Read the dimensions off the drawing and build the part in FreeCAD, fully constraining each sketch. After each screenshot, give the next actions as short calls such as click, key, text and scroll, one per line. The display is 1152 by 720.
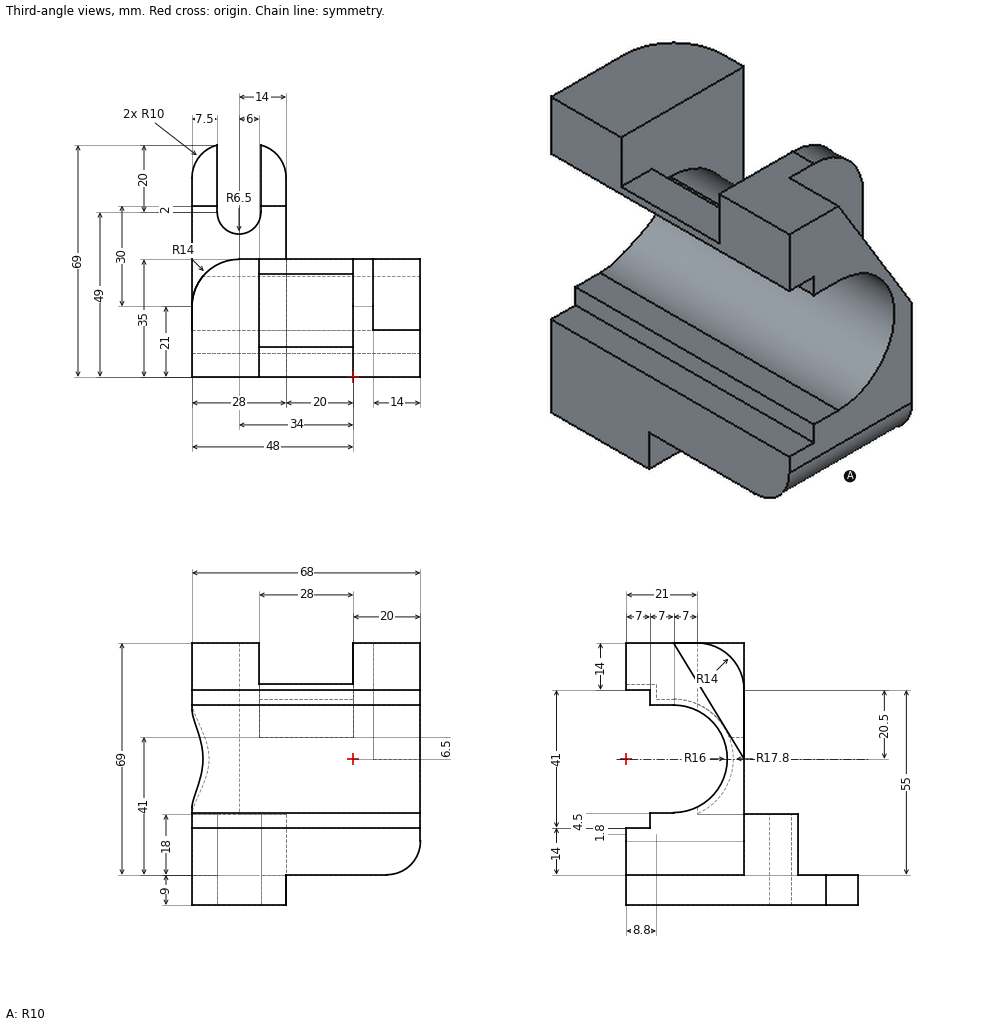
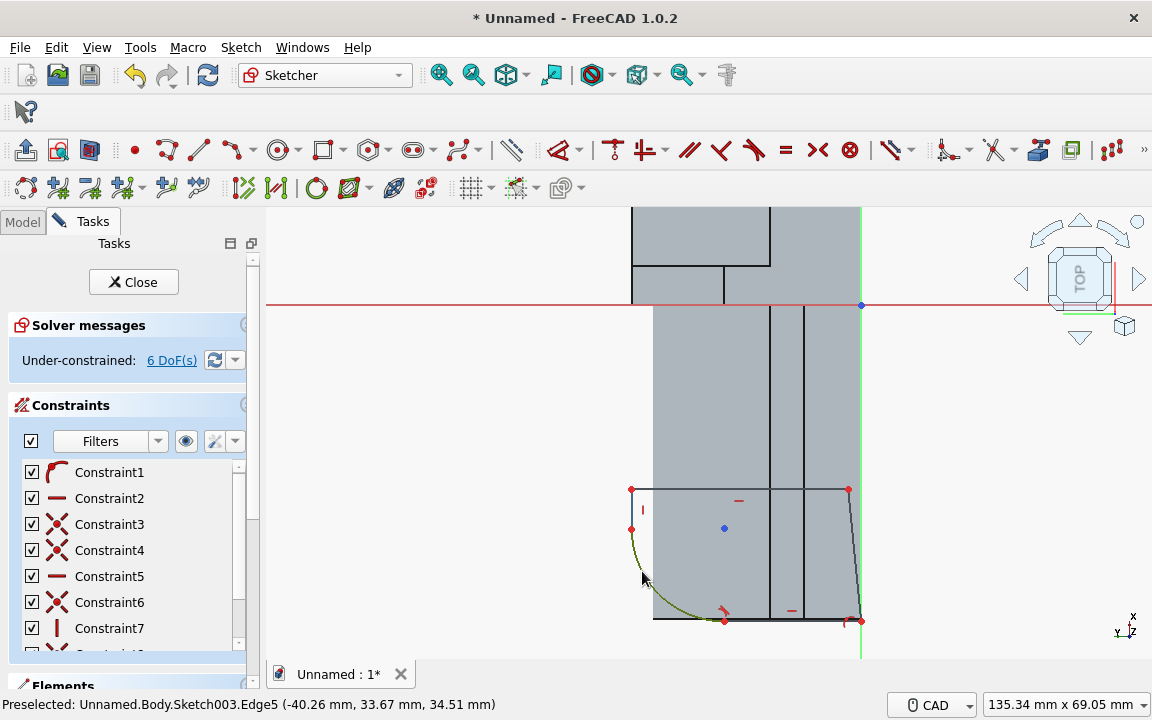
click(754, 150)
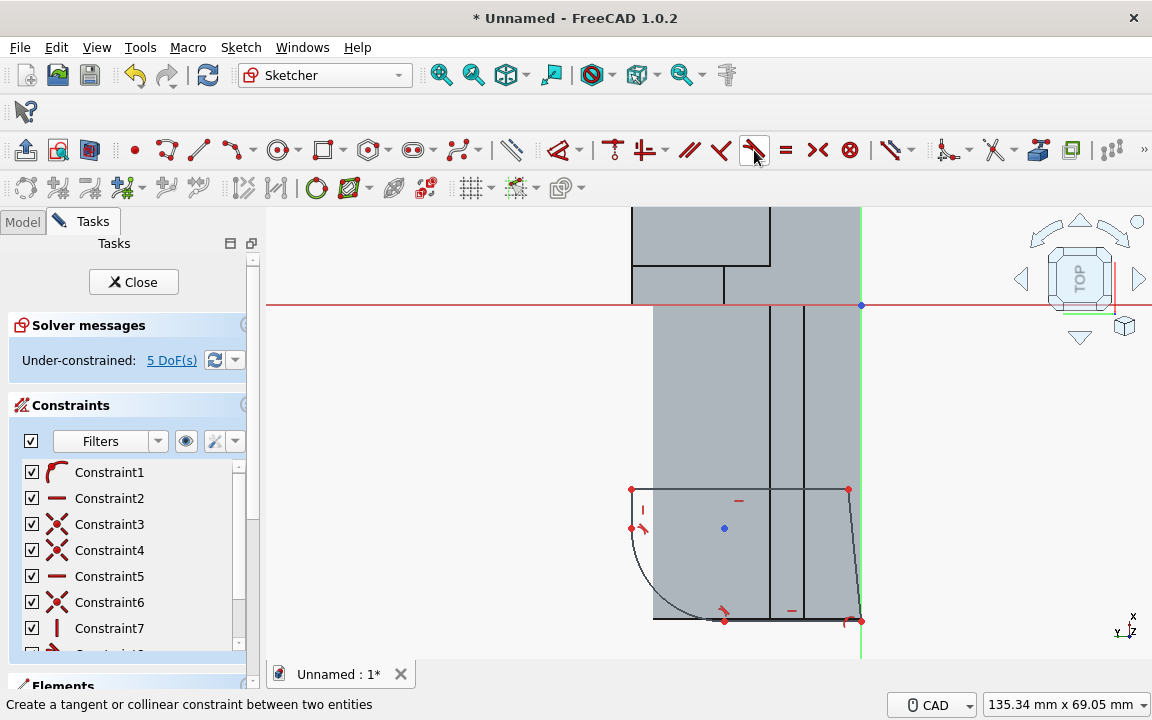
click(857, 582)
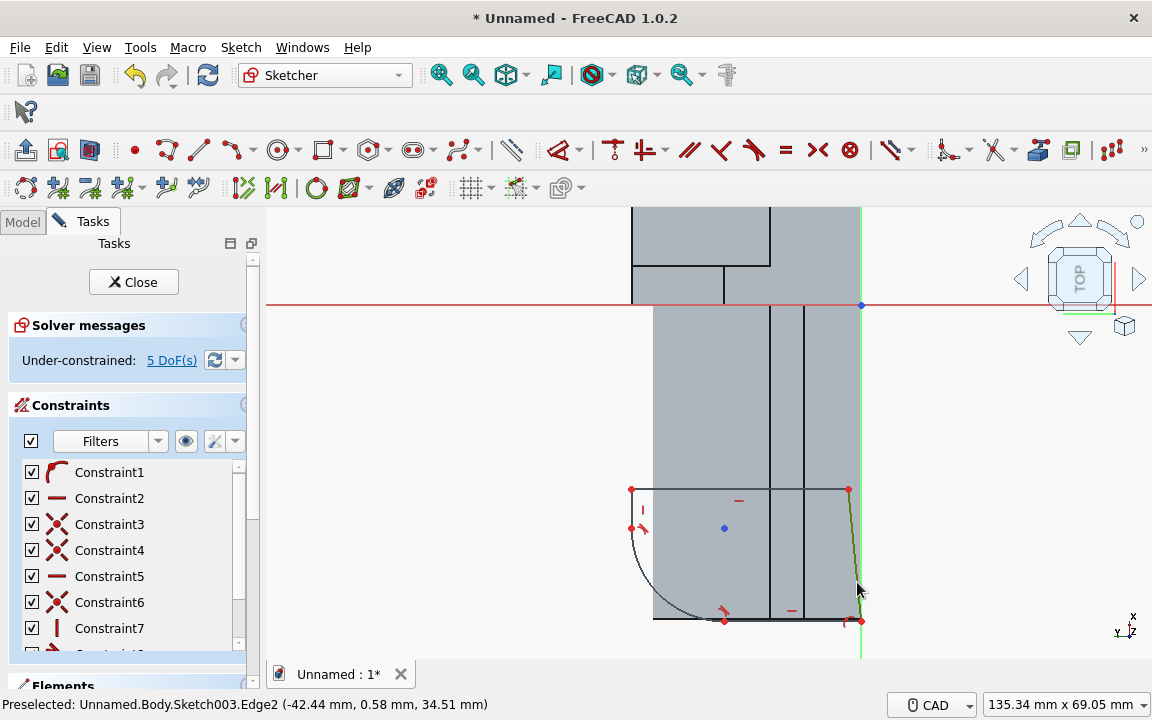
key(v)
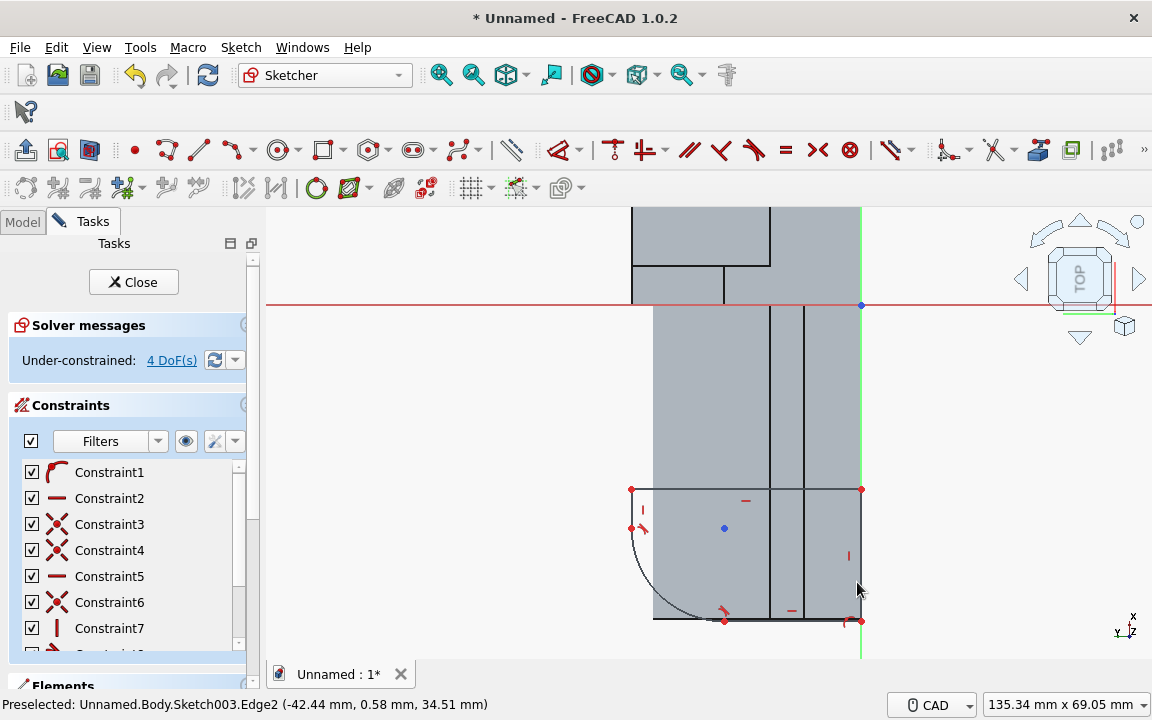
click(558, 150)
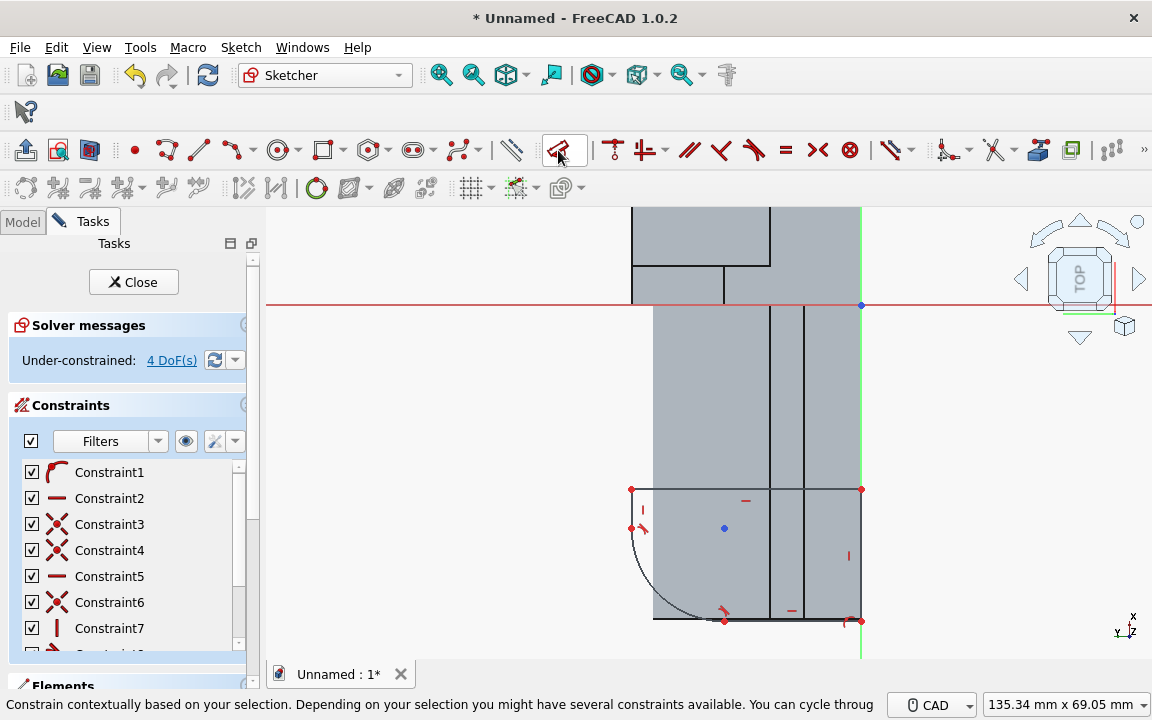
click(642, 571)
click(614, 586)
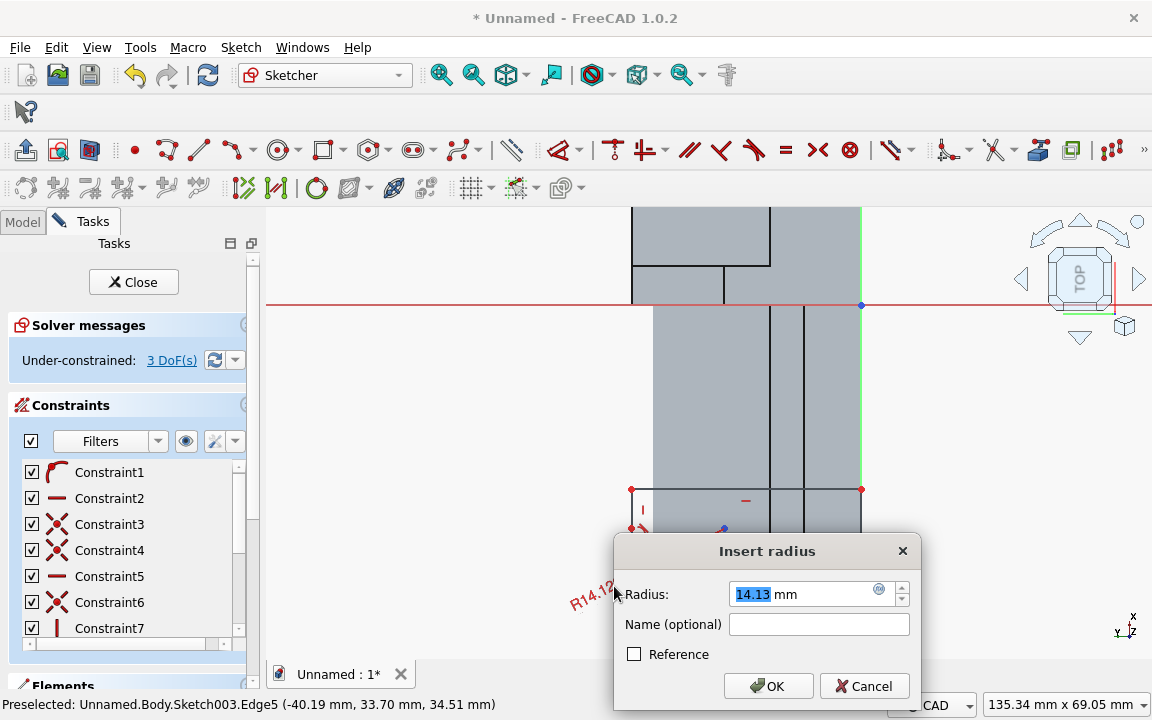
text(14)
key(Return)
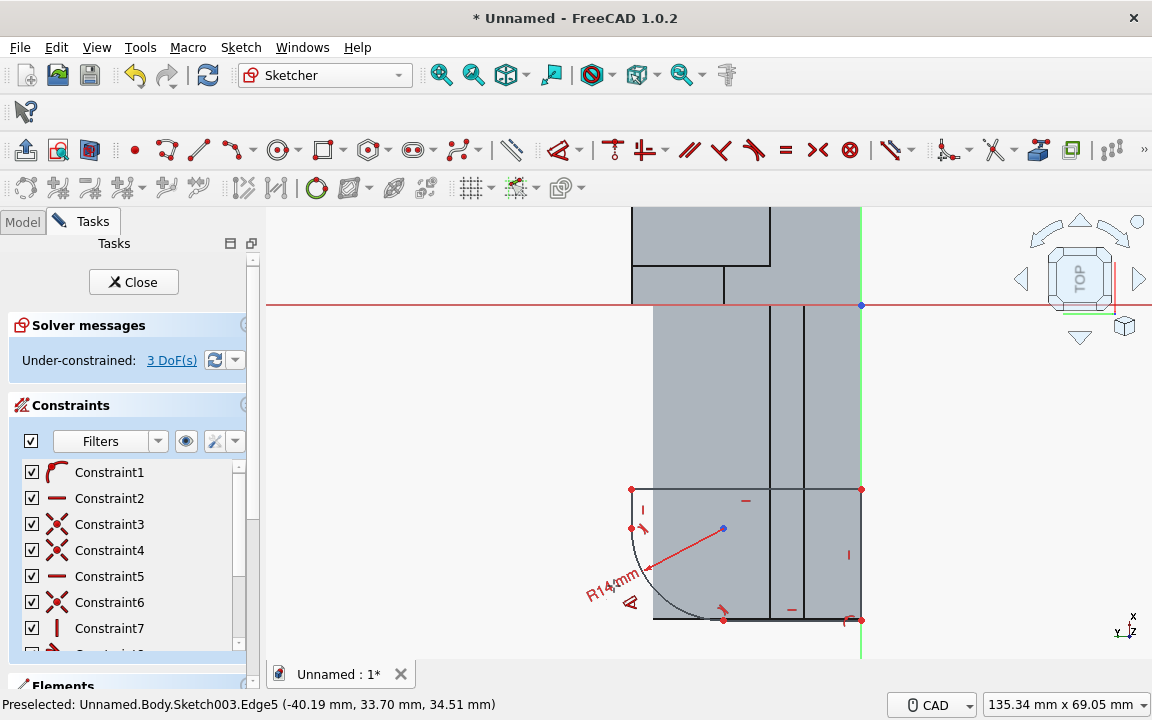
click(632, 501)
click(598, 509)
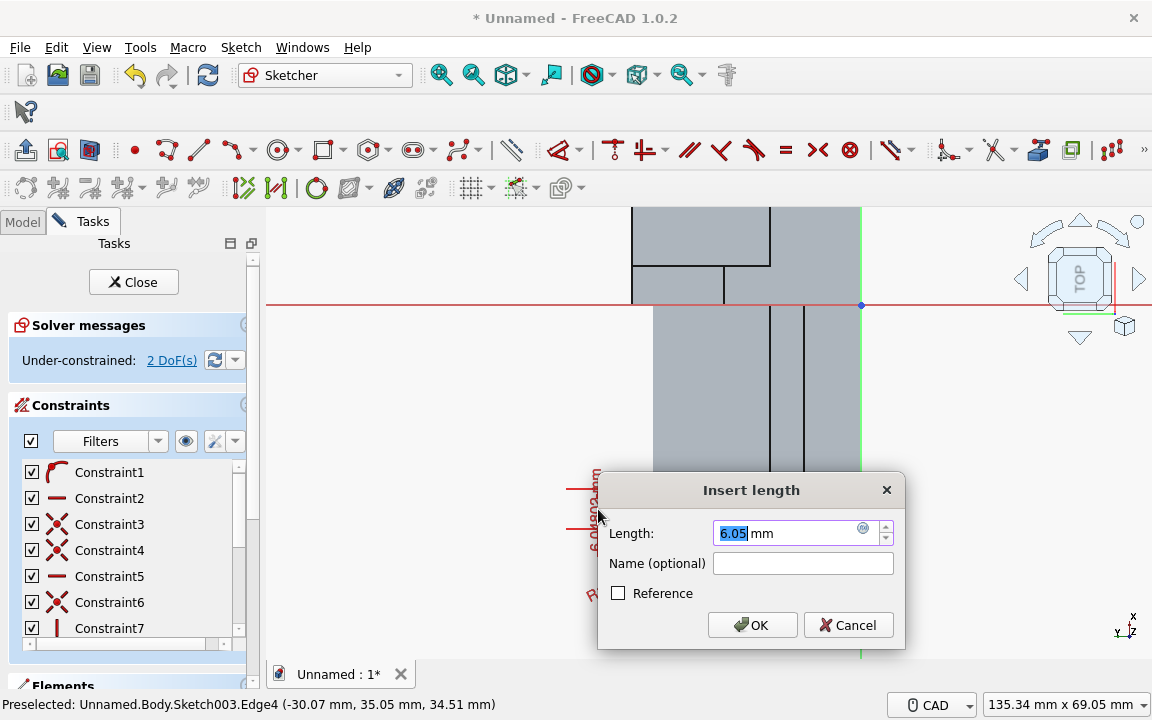
text(6)
key(Return)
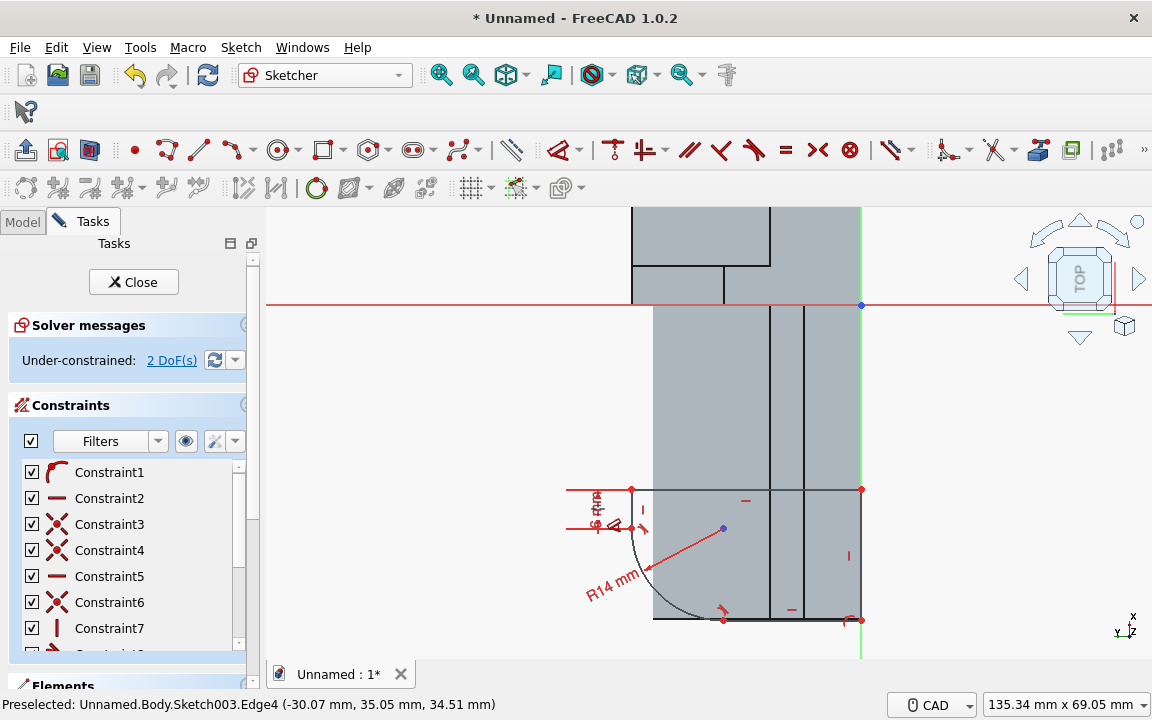
click(765, 621)
click(792, 587)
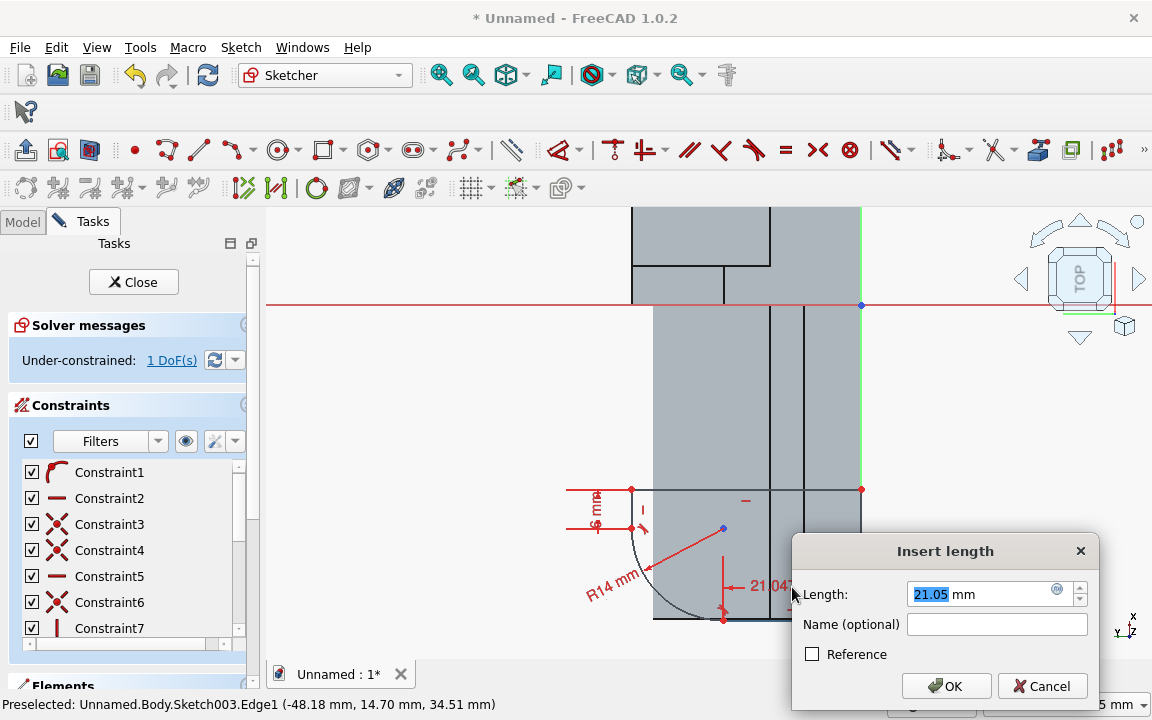
text(21)
key(Return)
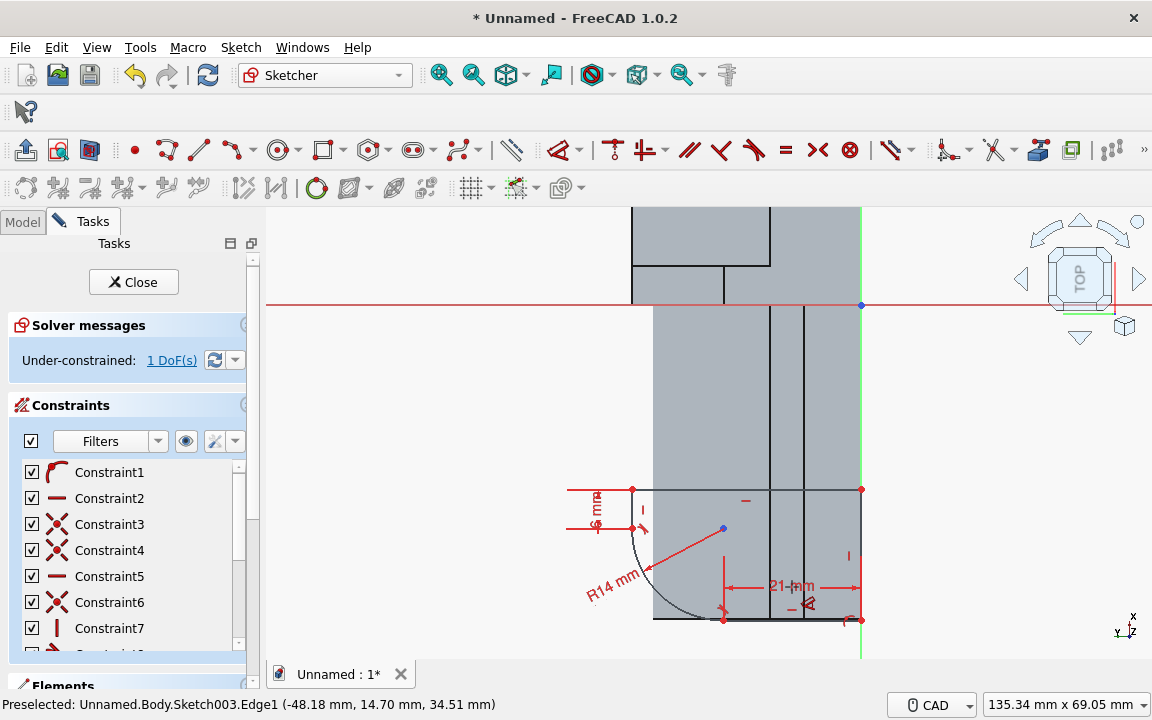
click(724, 621)
click(895, 463)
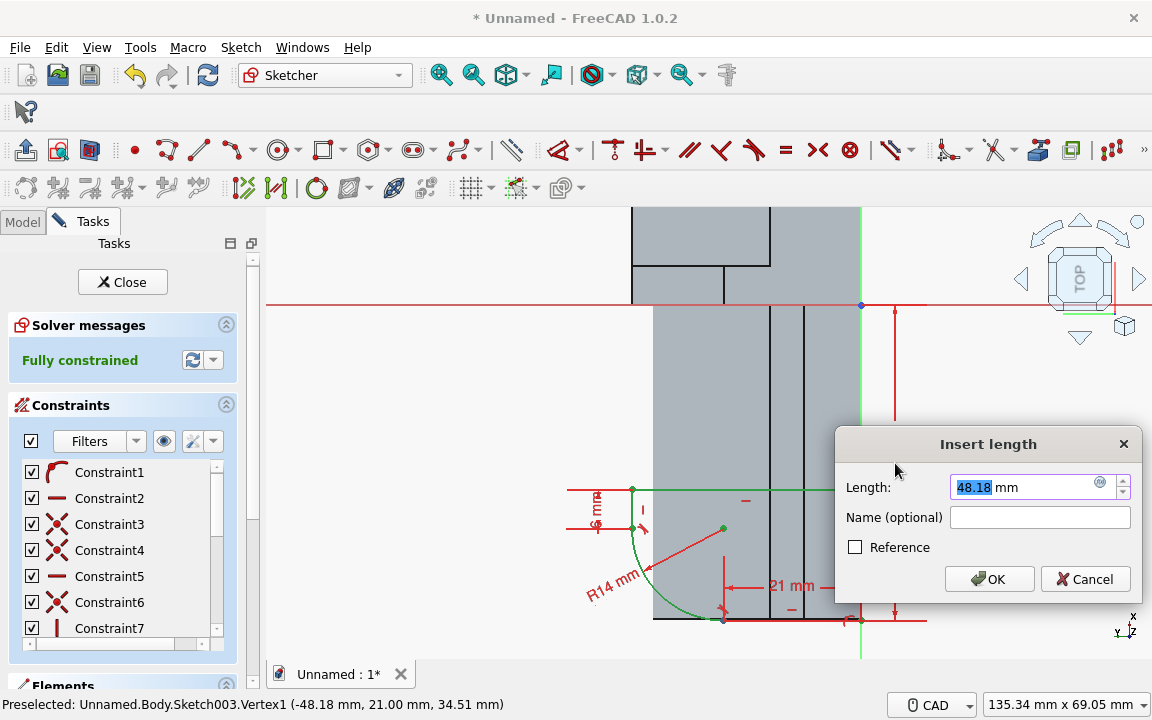
text(48)
key(Return)
key(Escape)